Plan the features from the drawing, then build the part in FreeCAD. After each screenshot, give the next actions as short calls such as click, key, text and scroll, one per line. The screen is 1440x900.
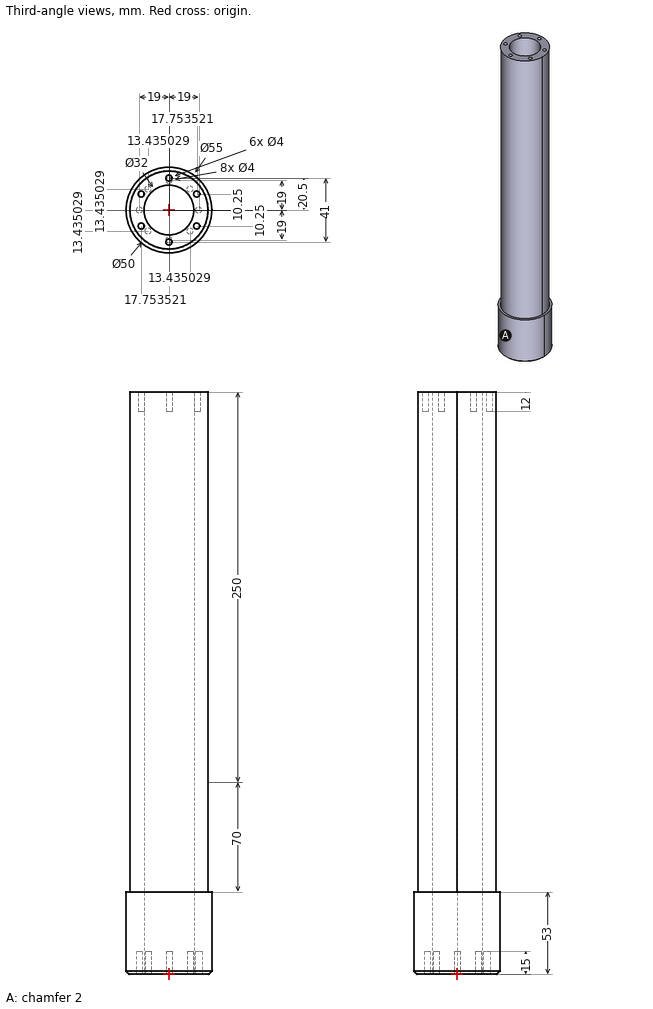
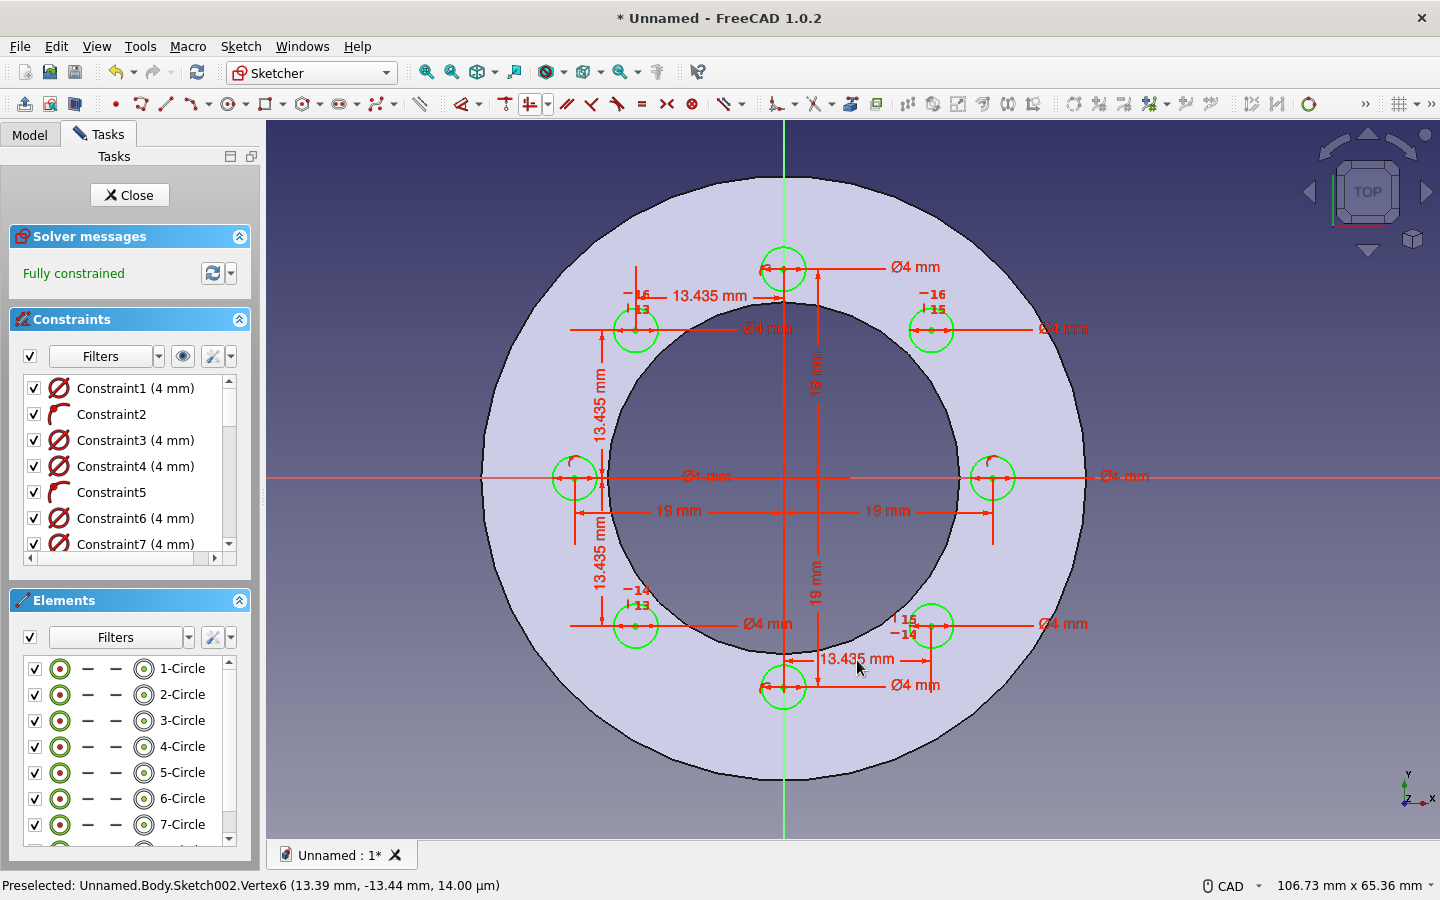
click(130, 195)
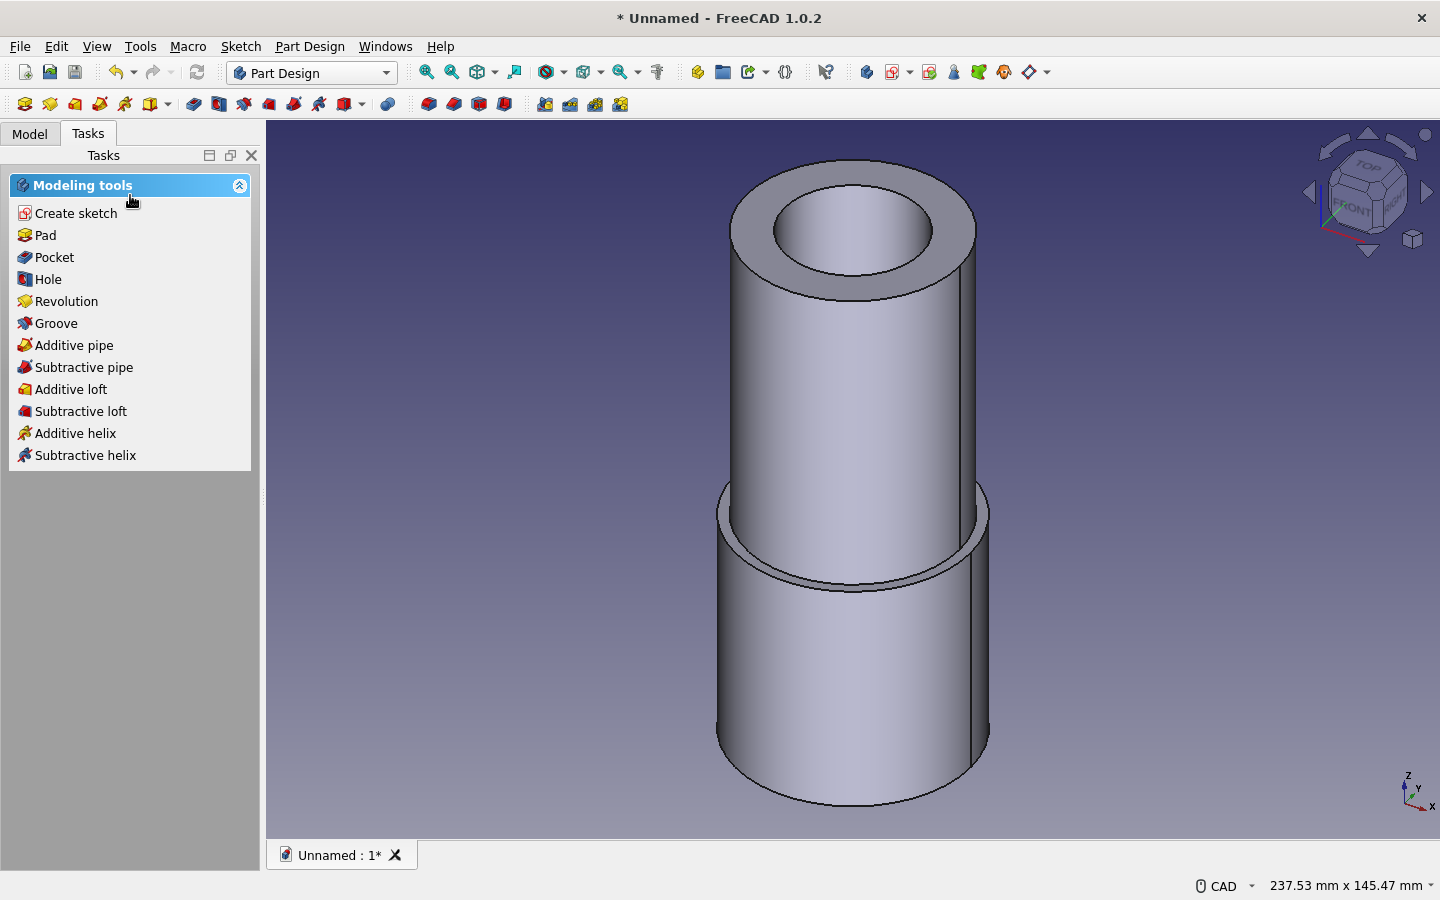
click(194, 104)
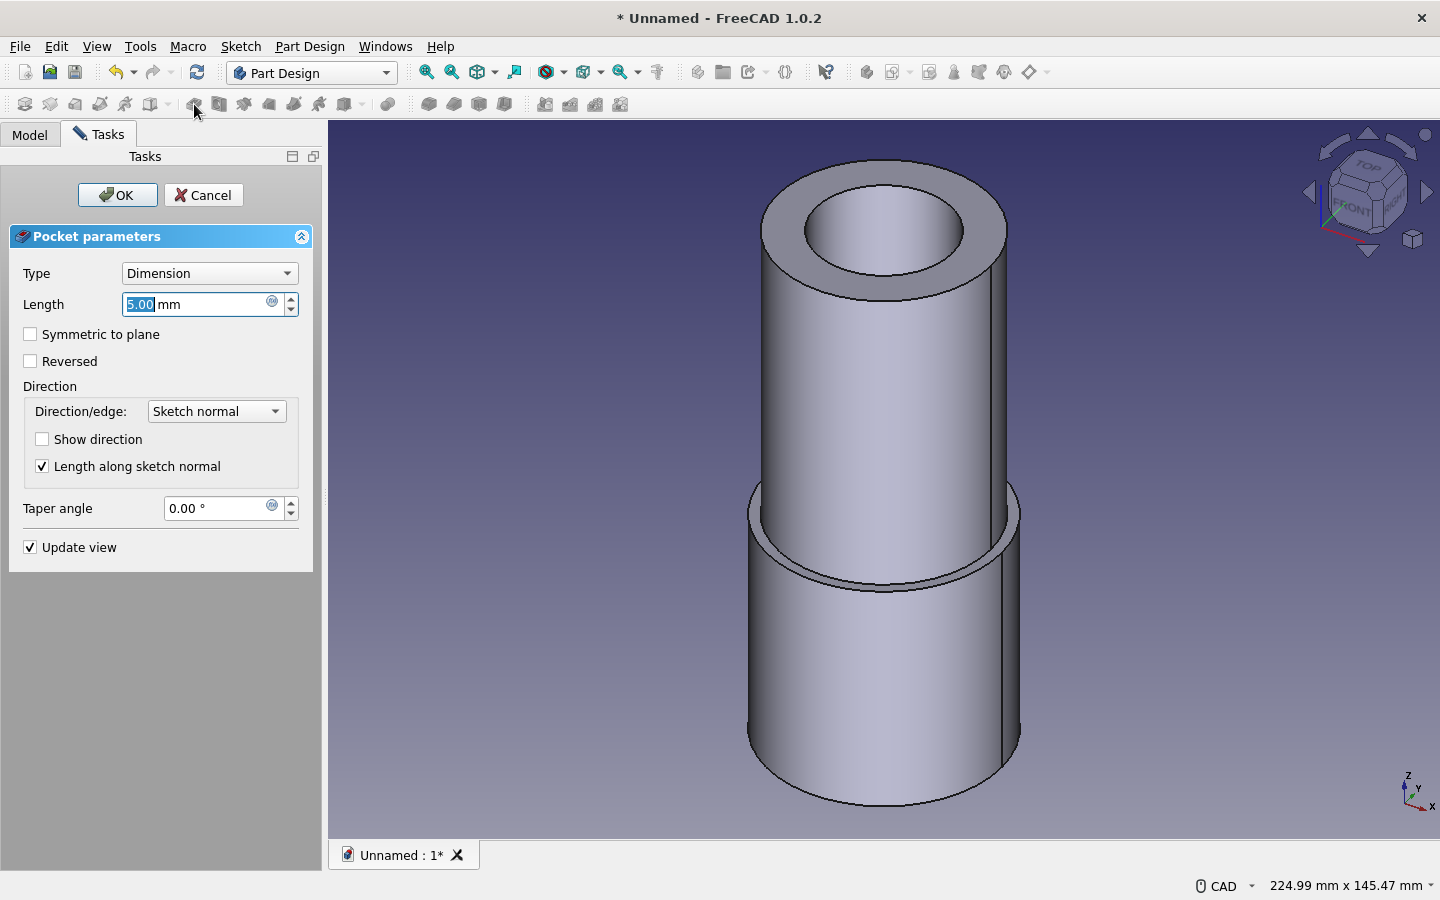
text(15)
key(Tab)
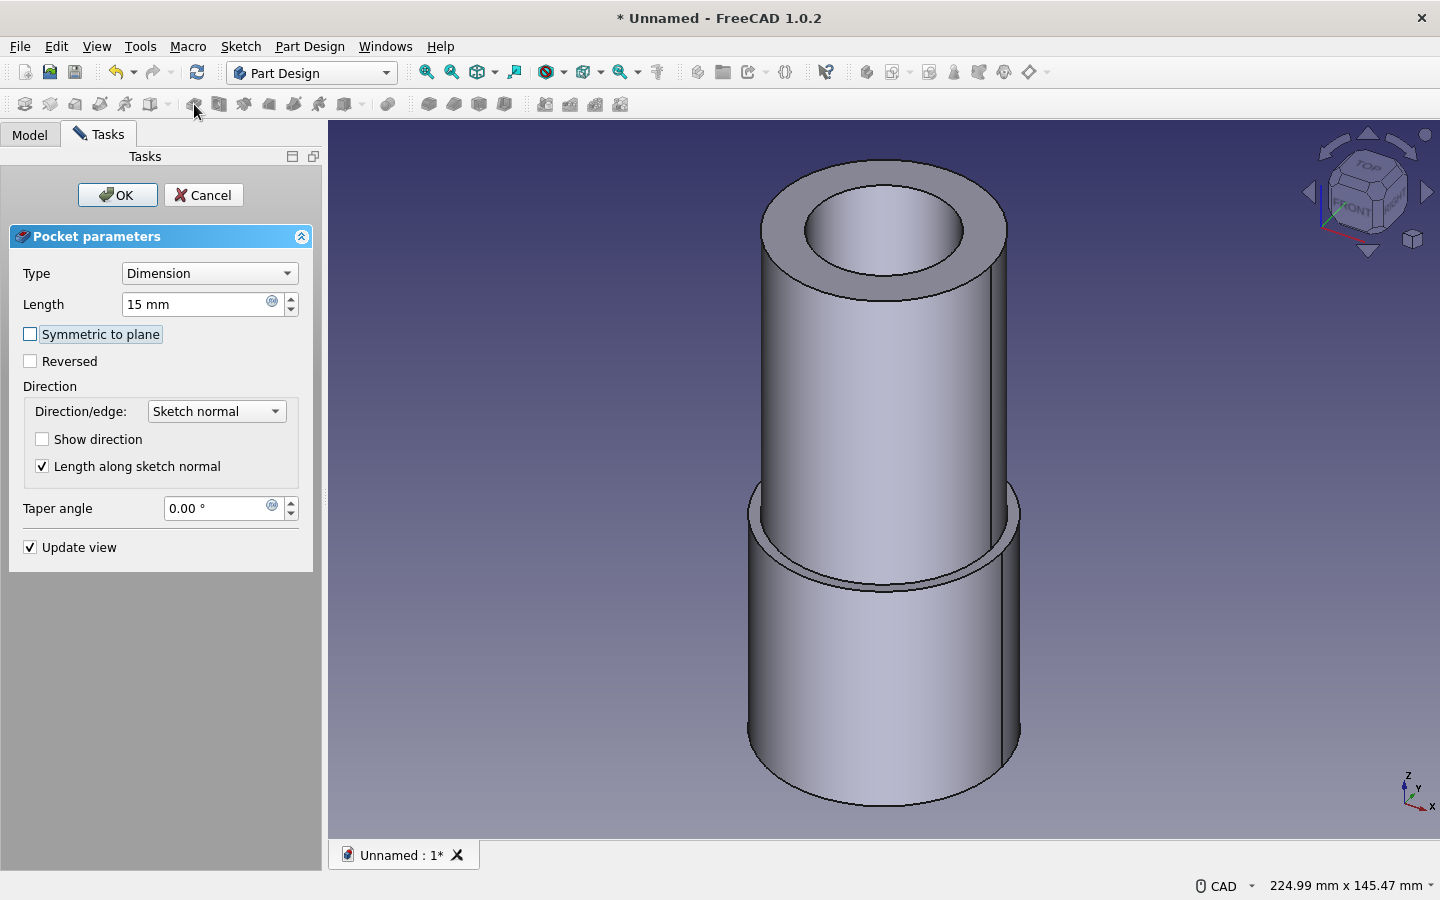
click(31, 361)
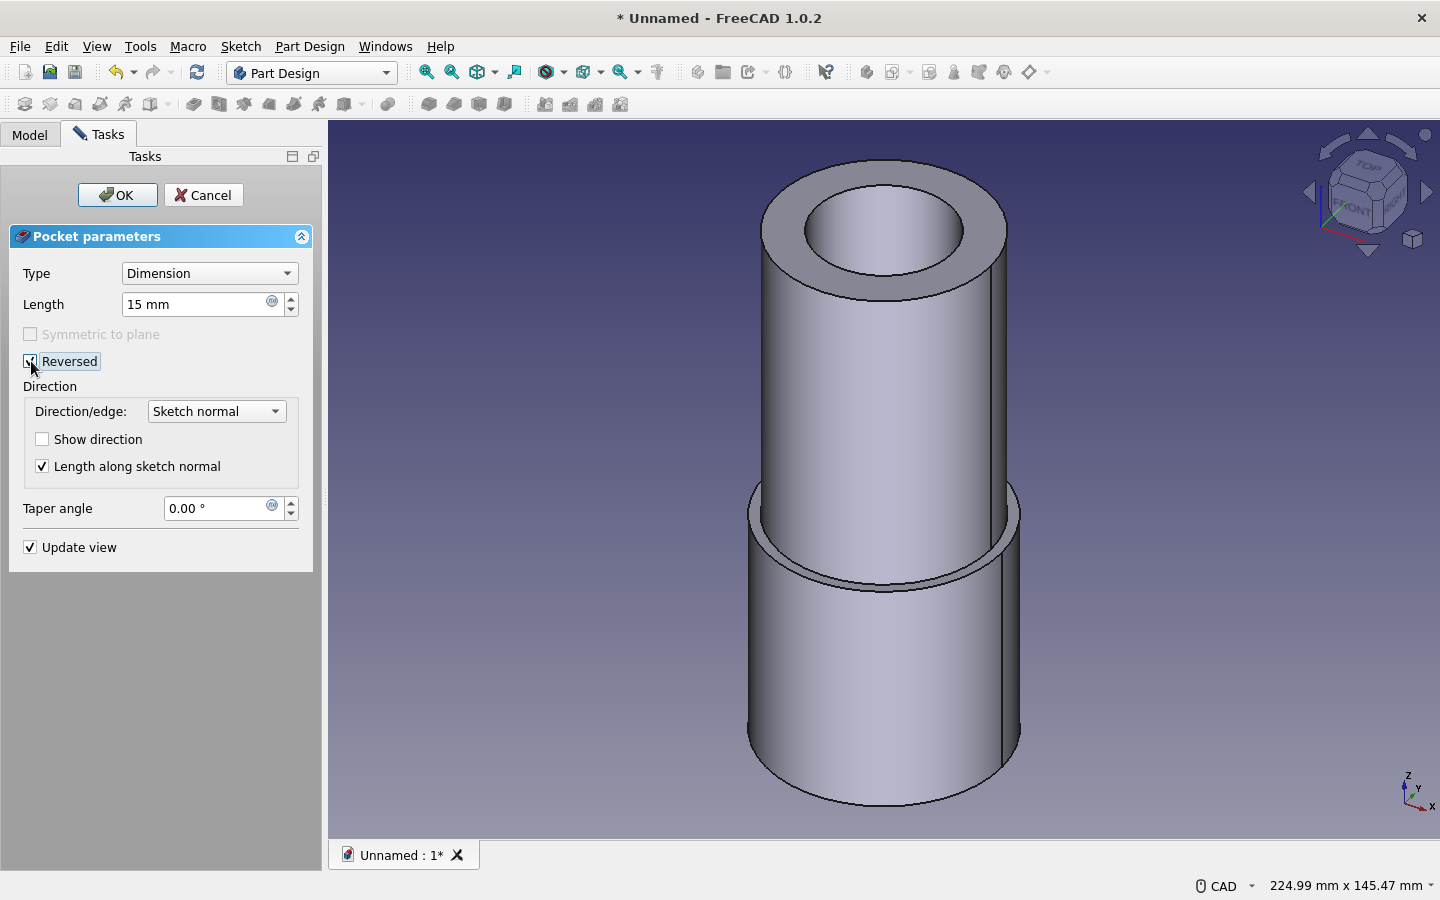
click(118, 195)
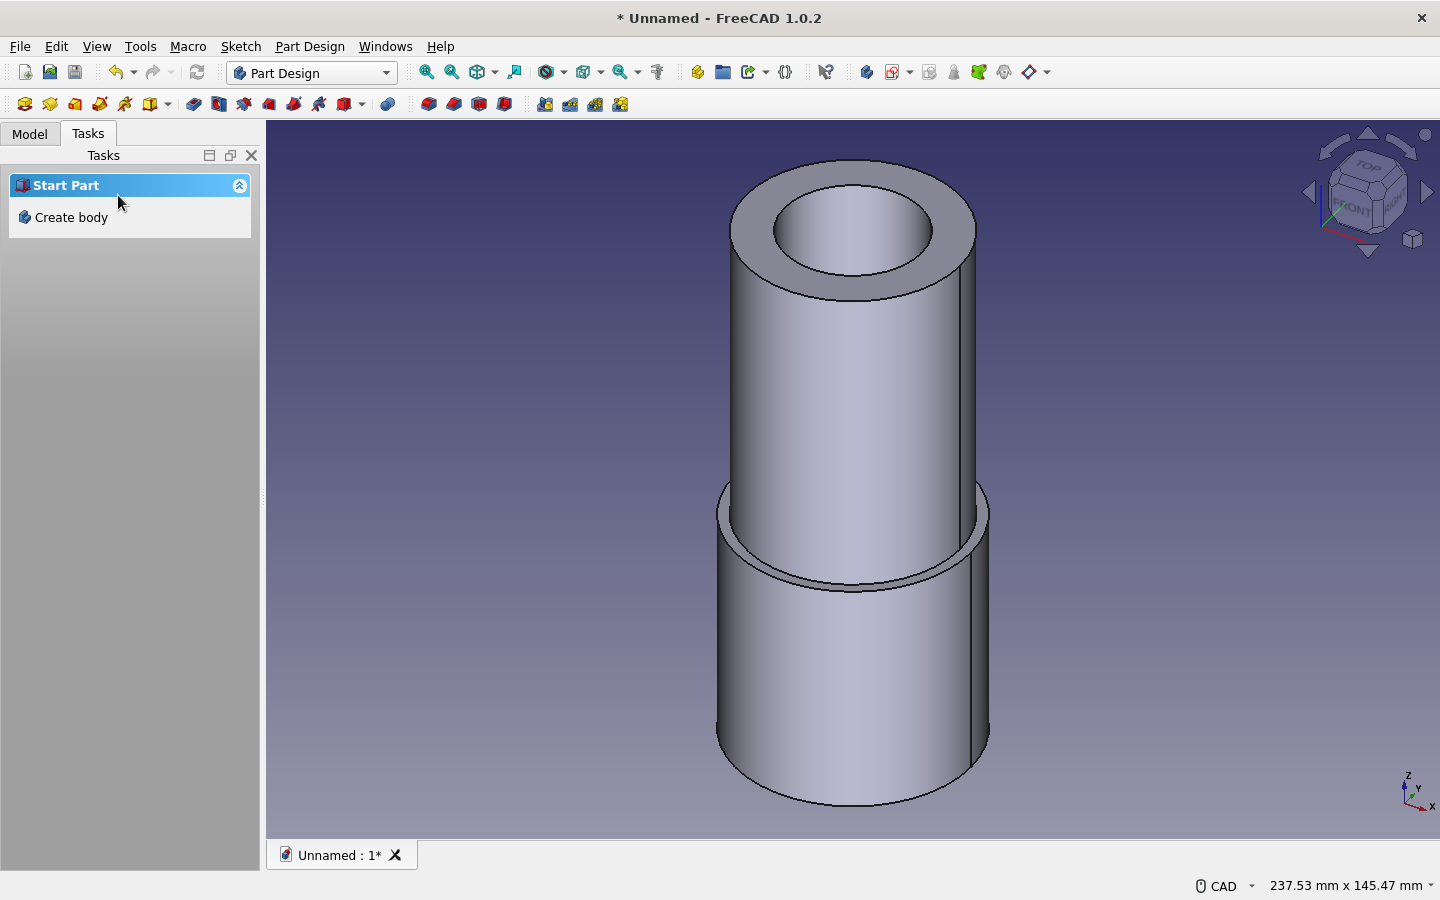
key(0)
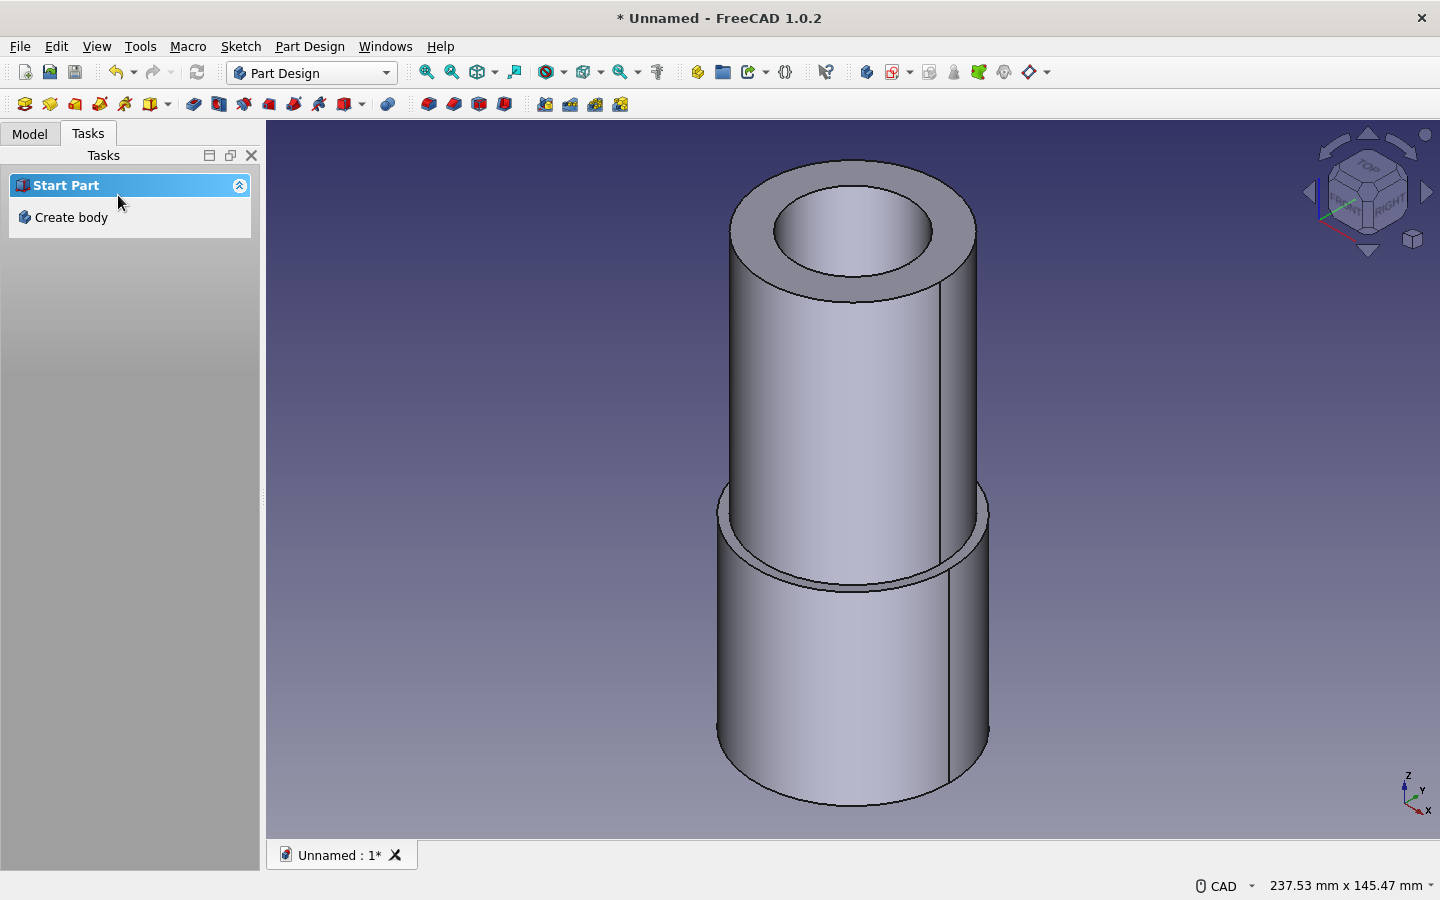
click(427, 72)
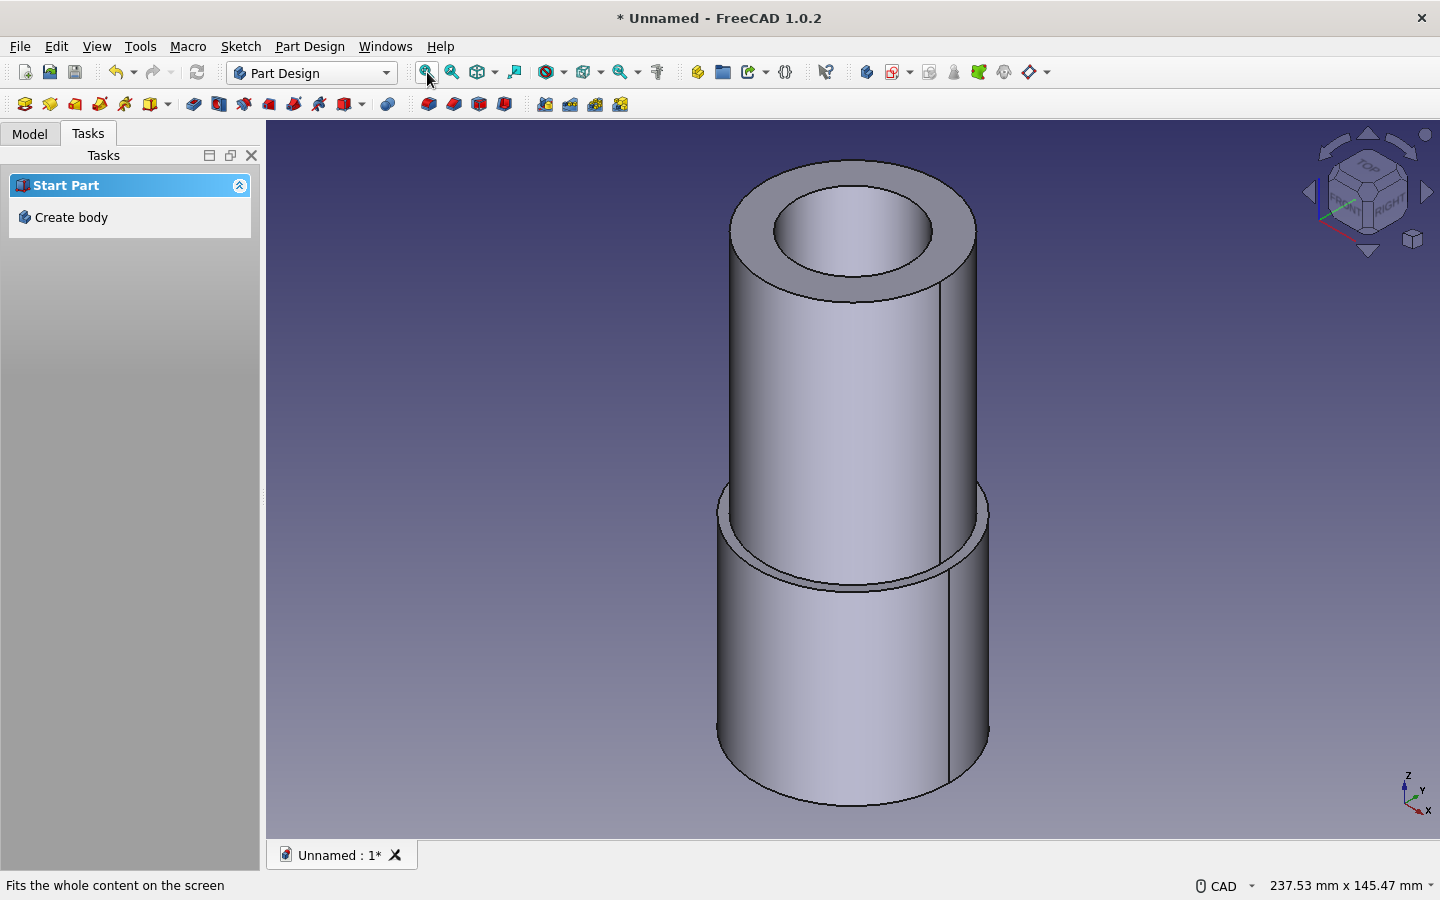
click(965, 771)